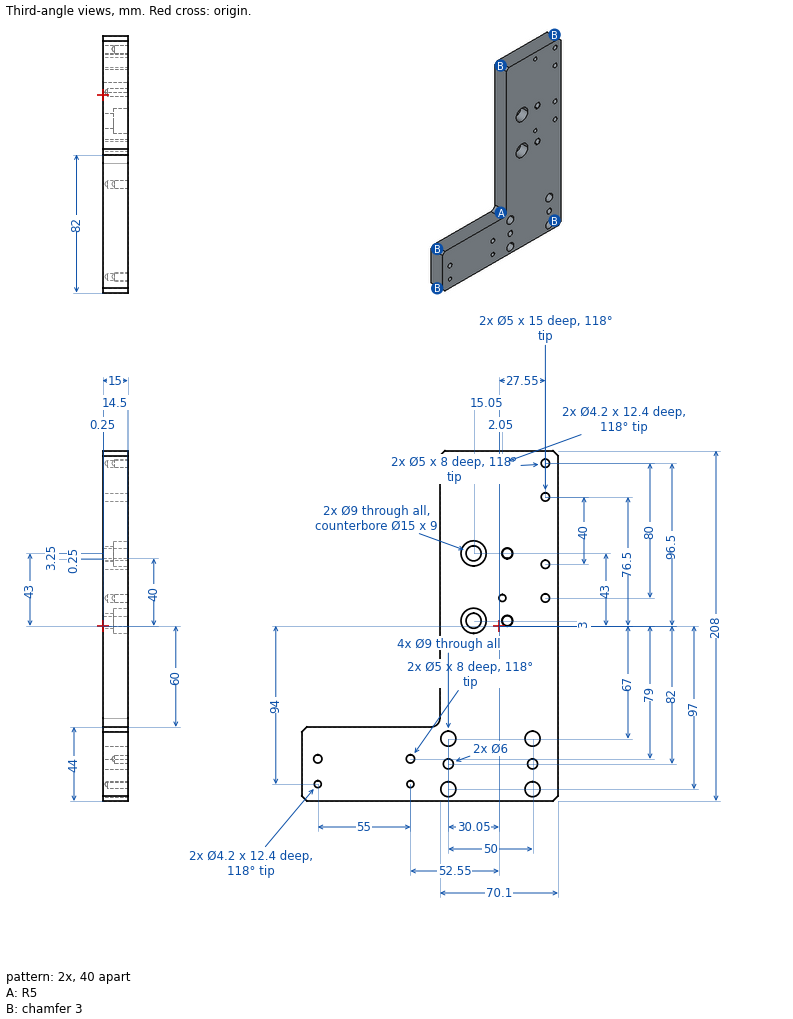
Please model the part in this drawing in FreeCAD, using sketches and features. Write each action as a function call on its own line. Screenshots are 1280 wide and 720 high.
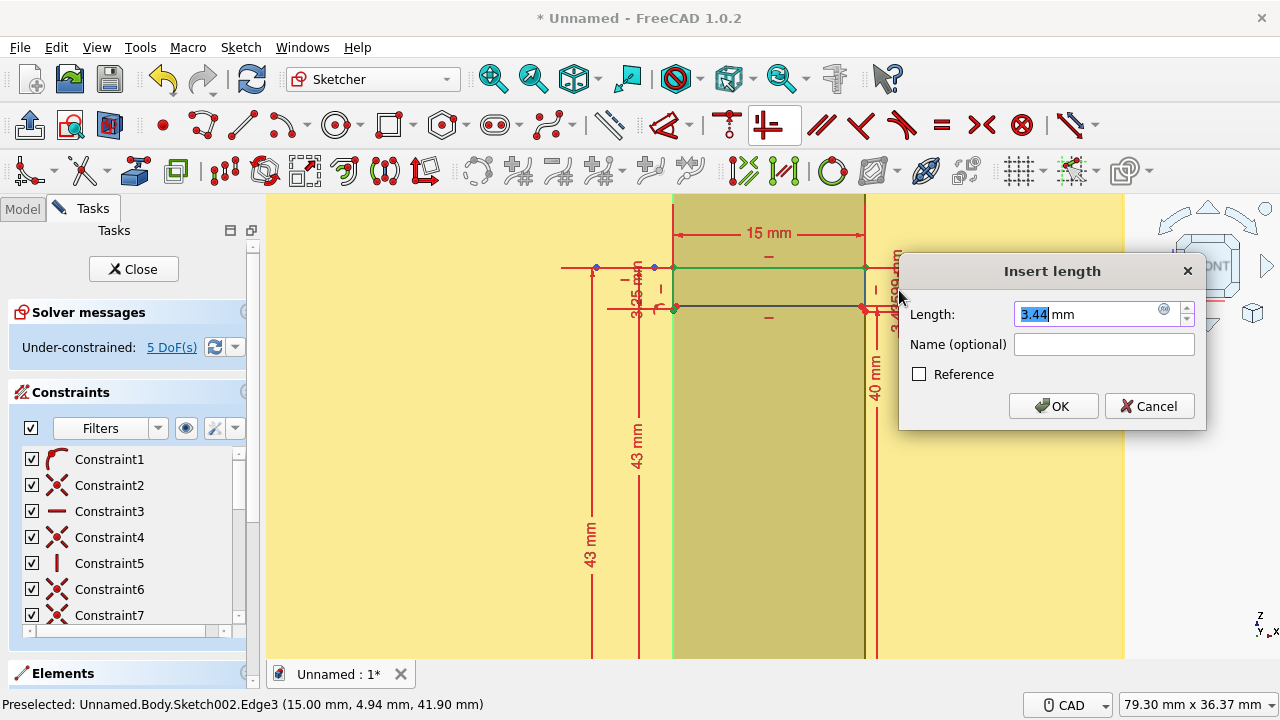
text(3.25)
key(Return)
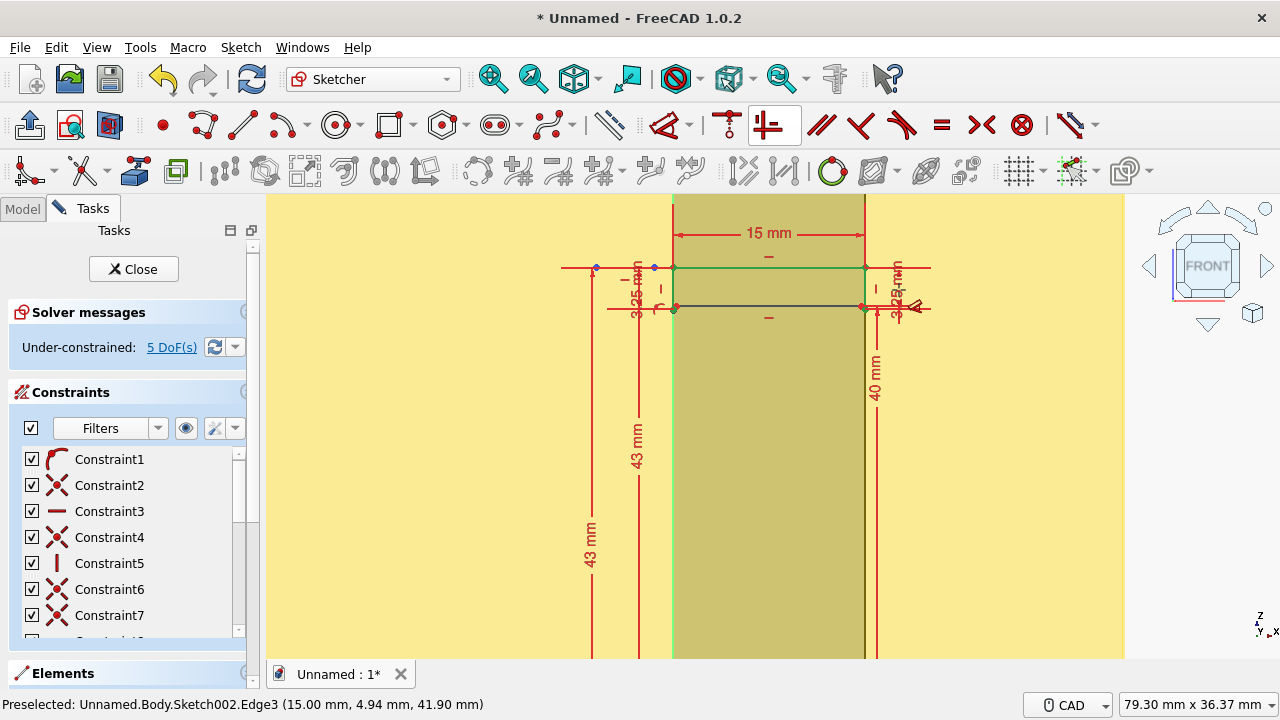
click(806, 306)
click(769, 340)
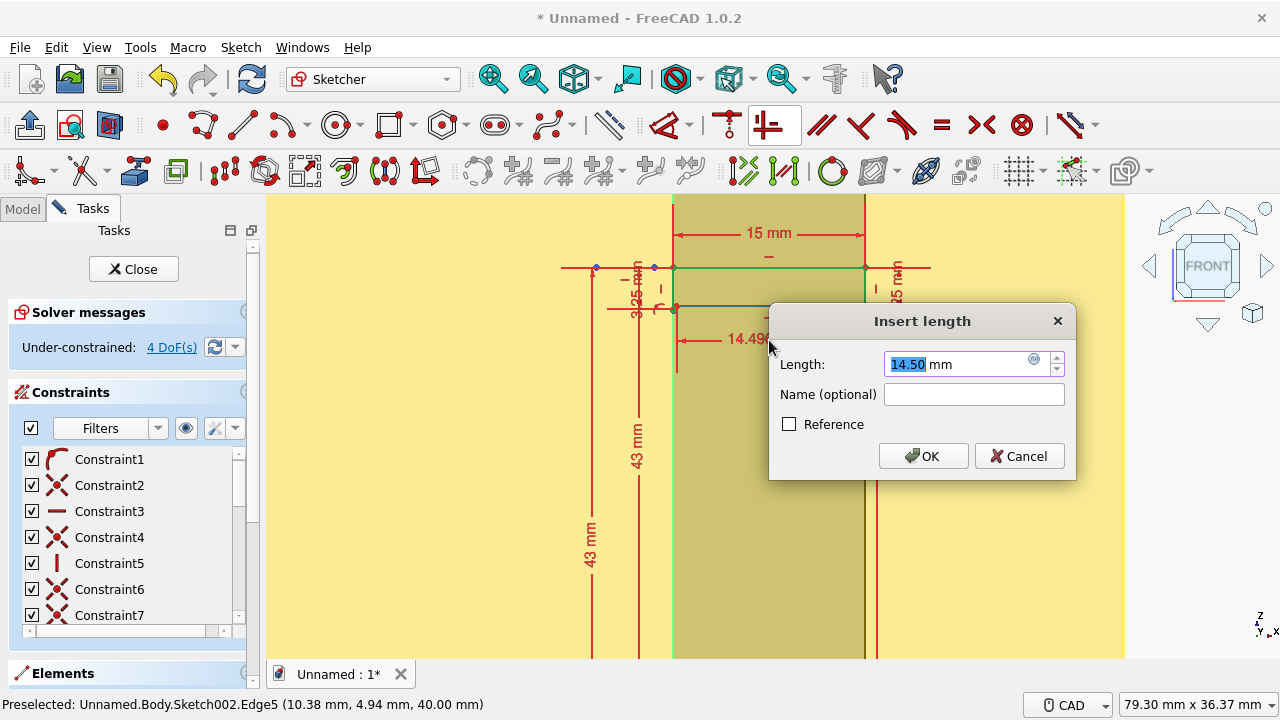
text(14.5)
key(Return)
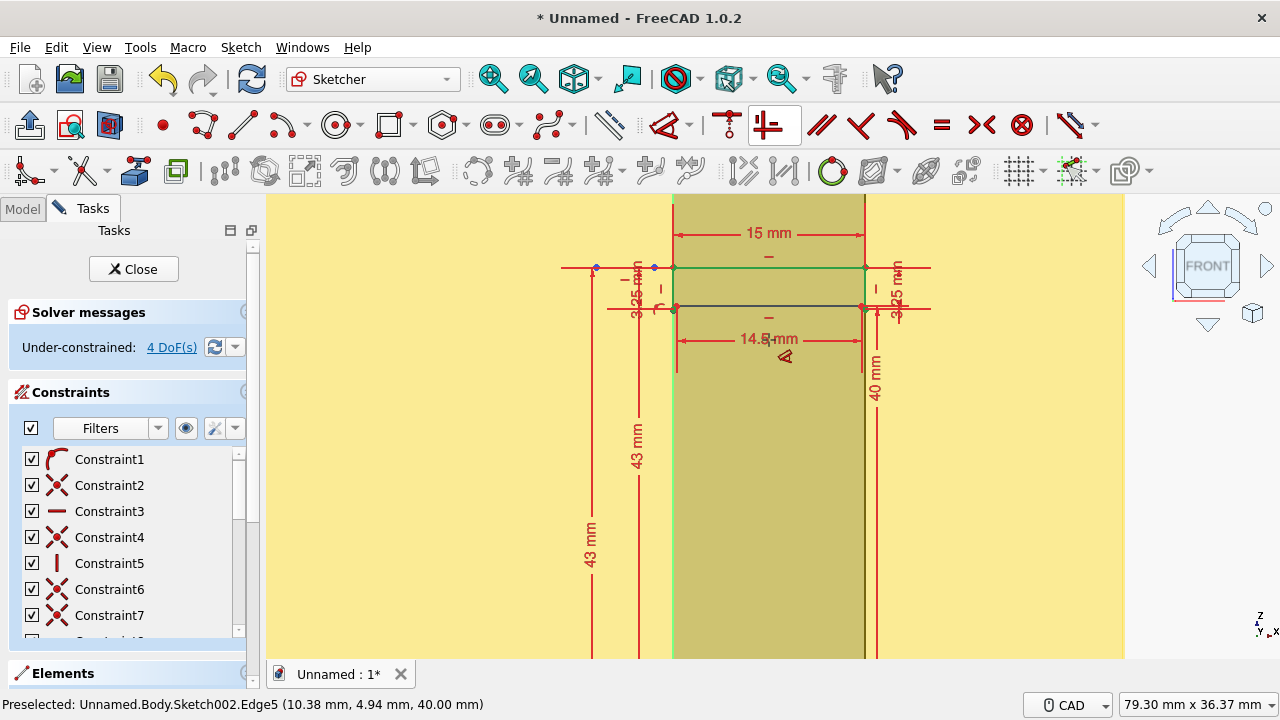
scroll(677, 306, up, 13)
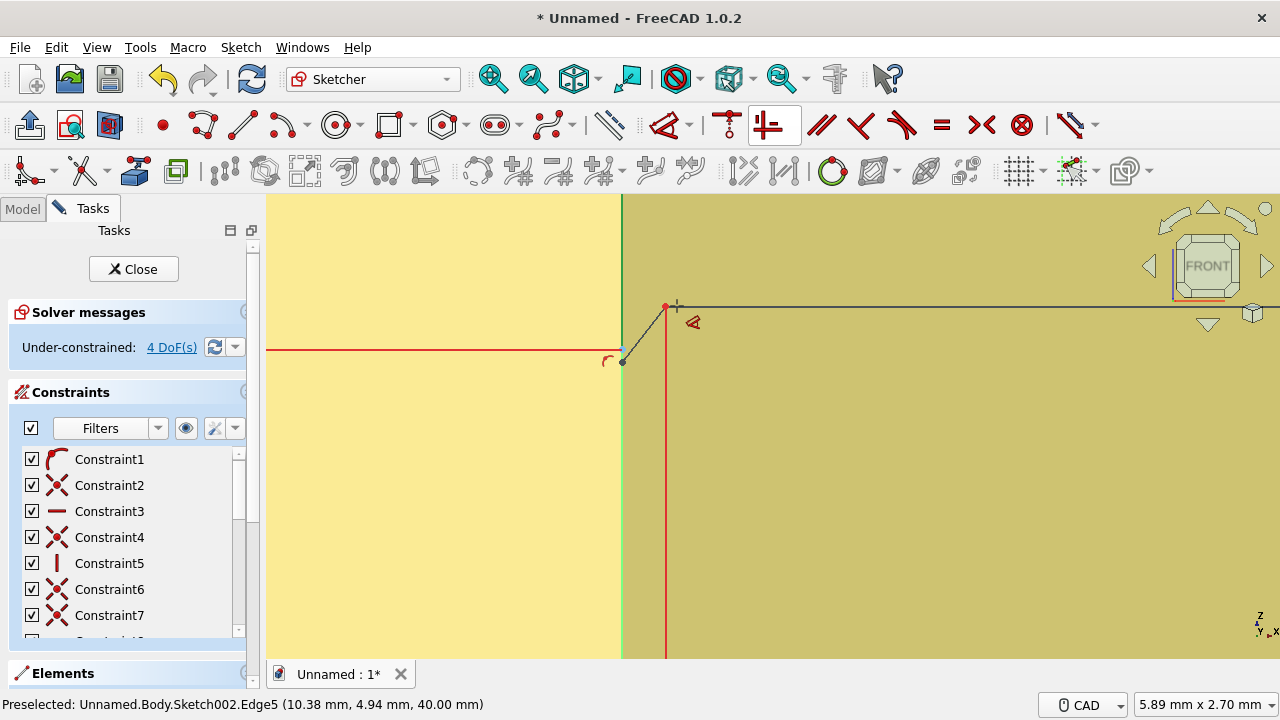
click(666, 307)
click(644, 273)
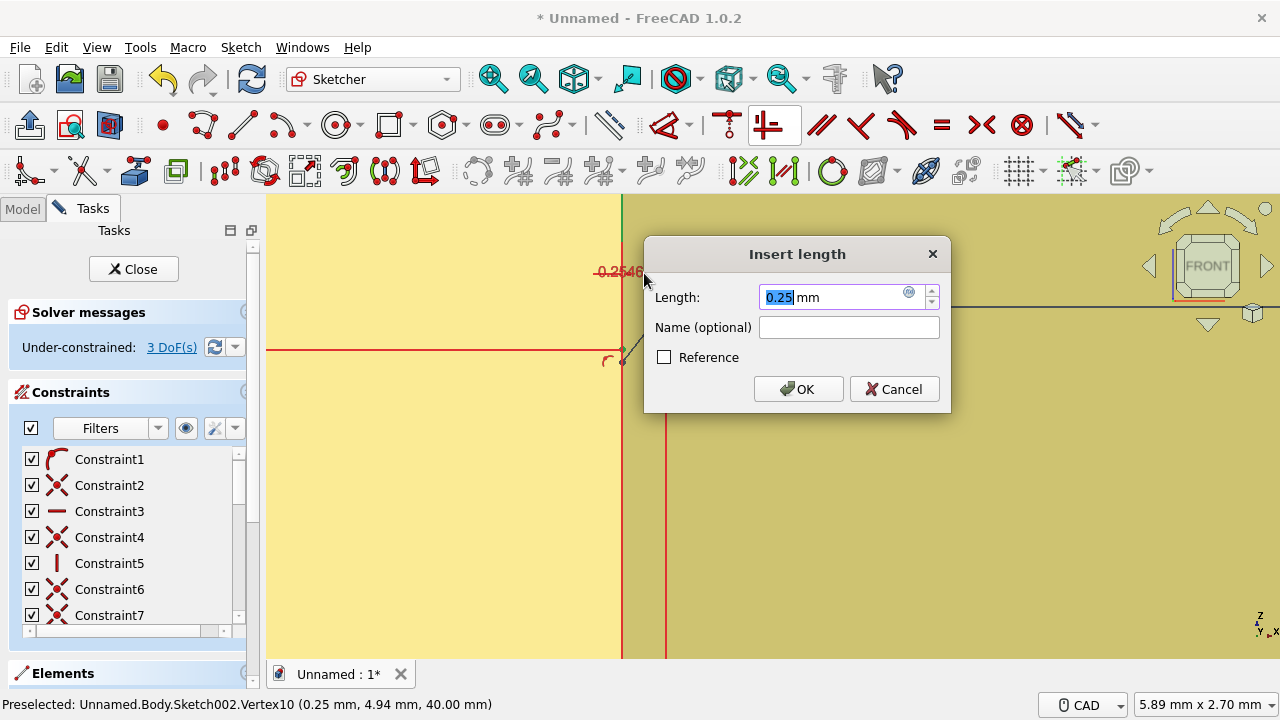
text(0.25)
key(Return)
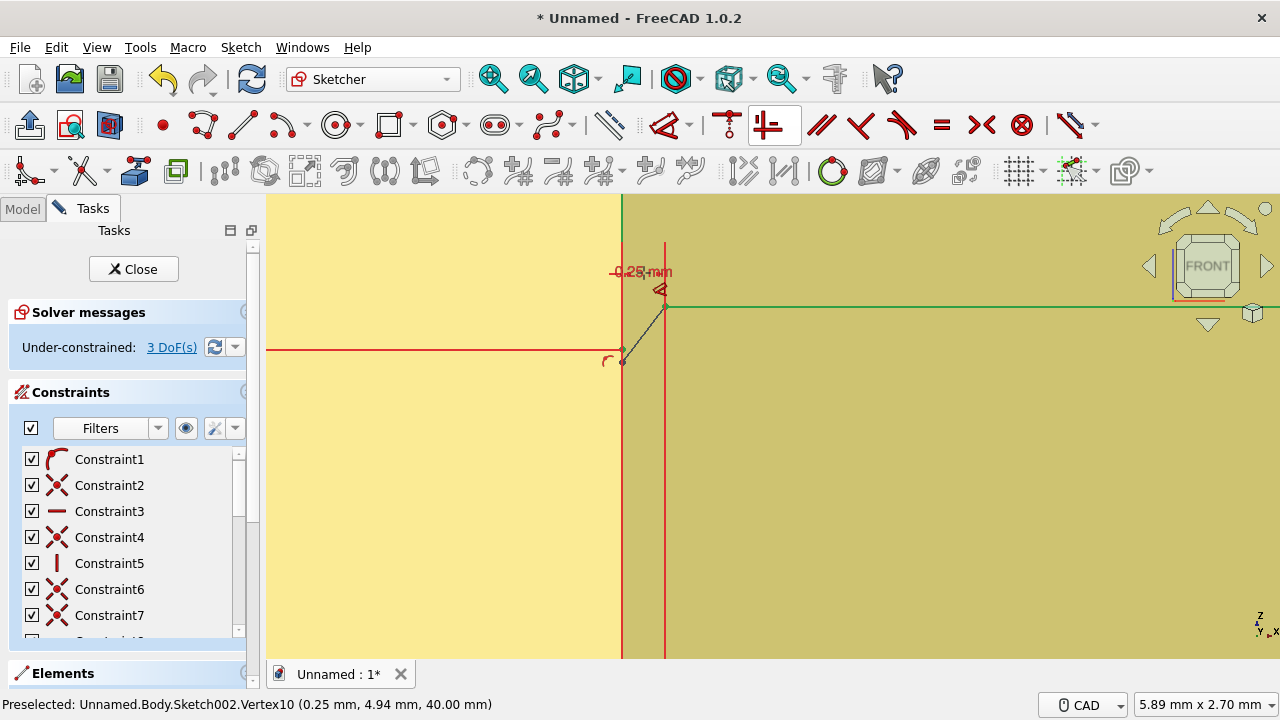
click(652, 323)
click(588, 335)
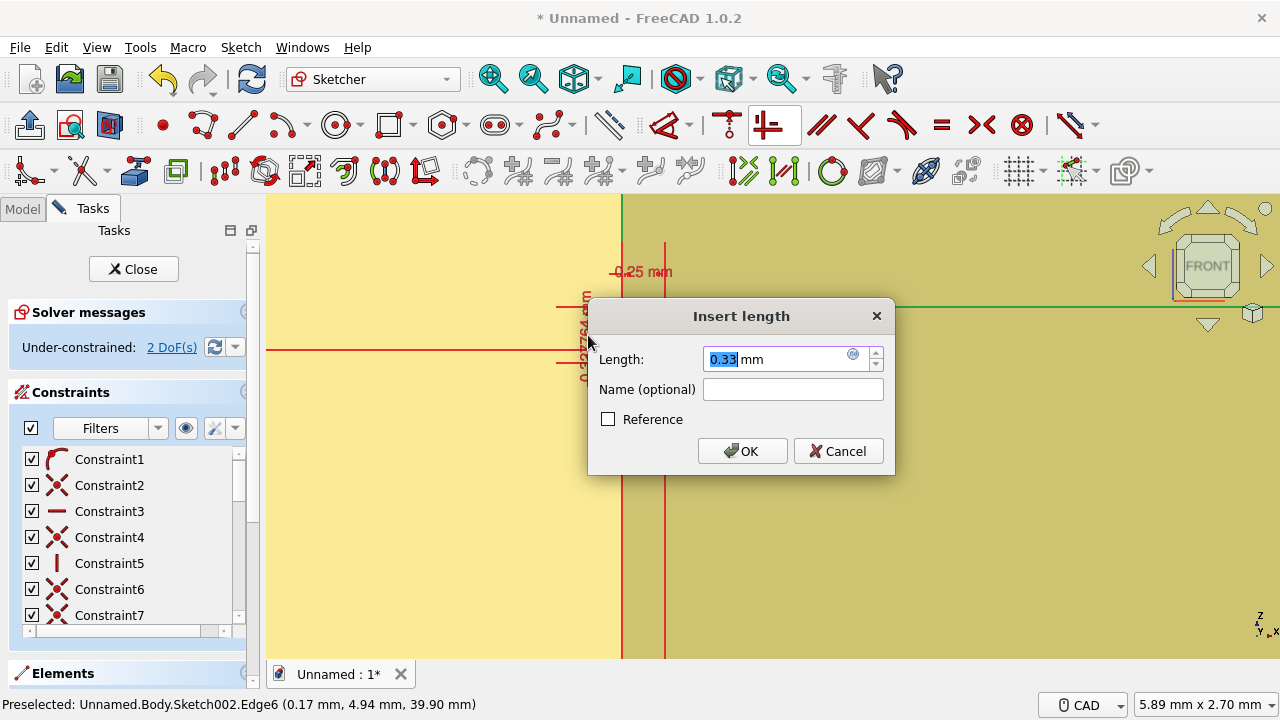
text(0.25)
key(Return)
key(Escape)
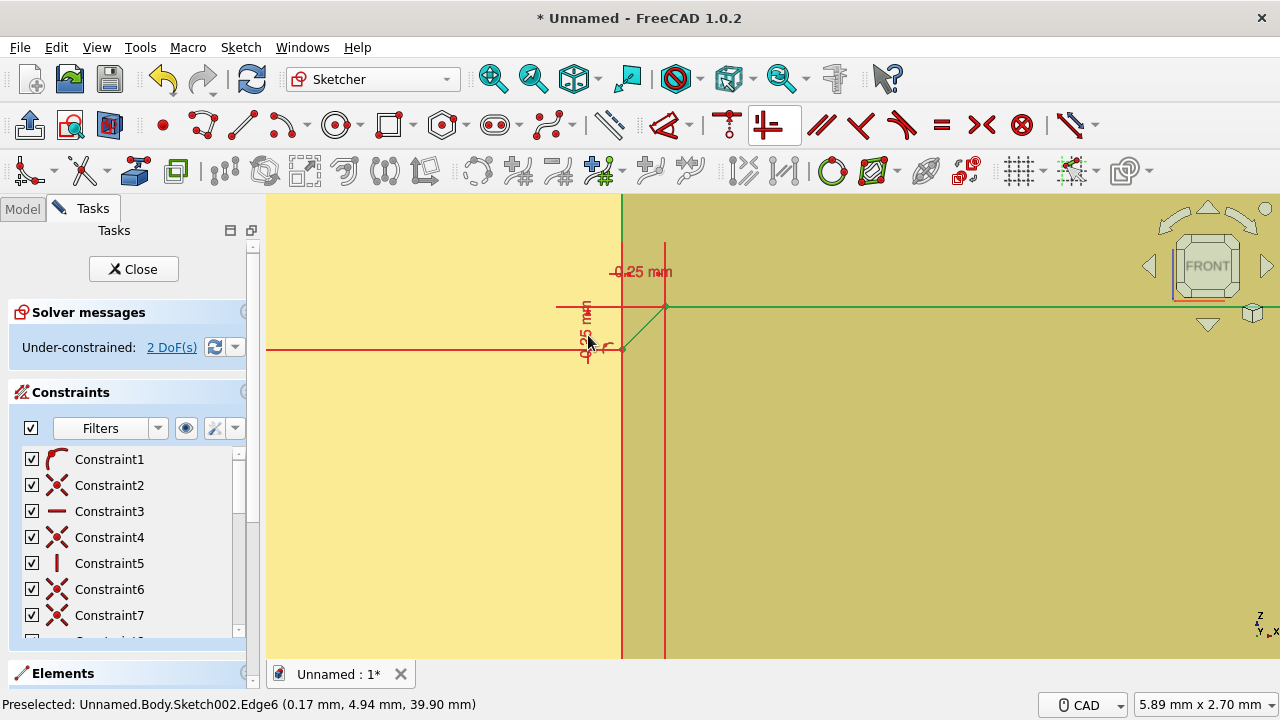
click(134, 269)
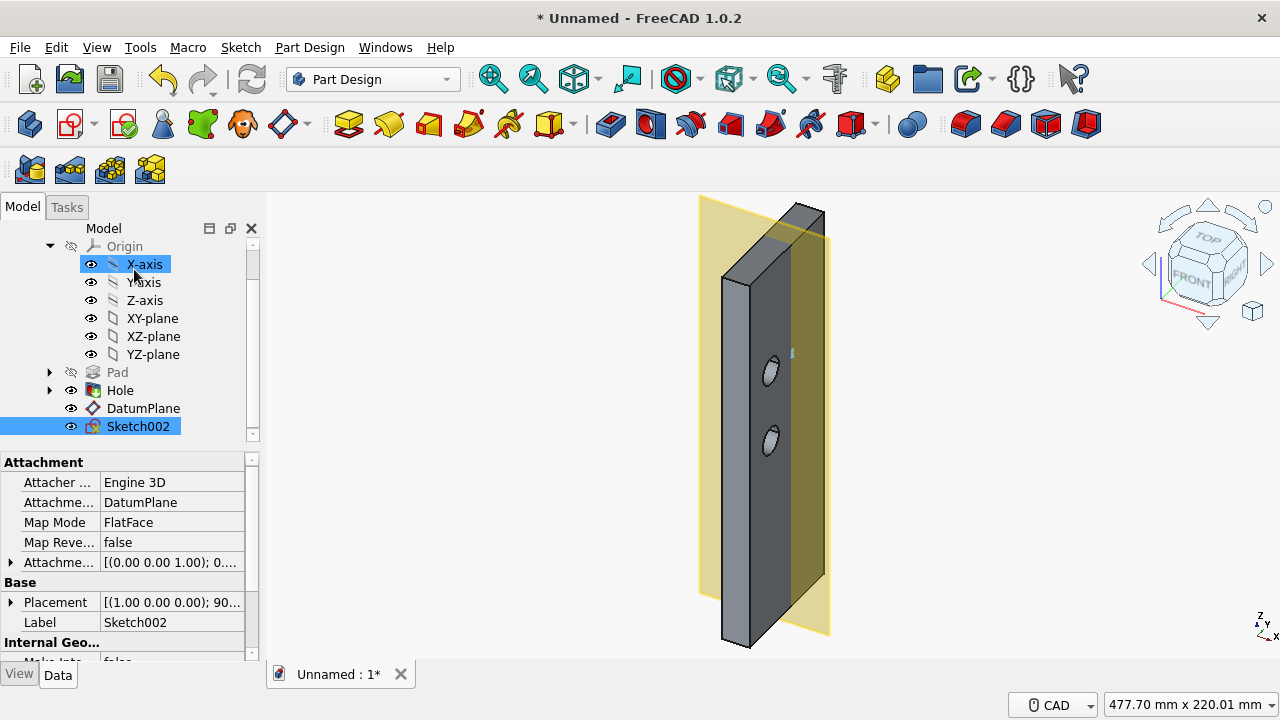
click(692, 124)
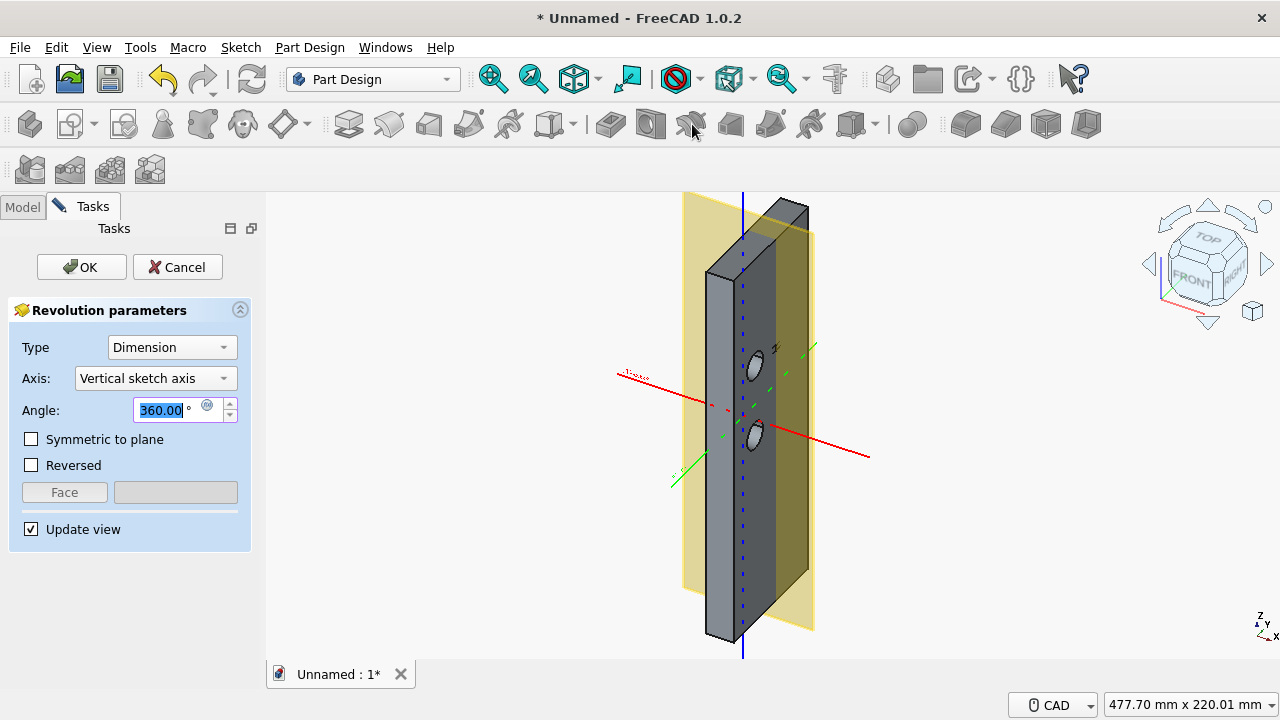
click(156, 378)